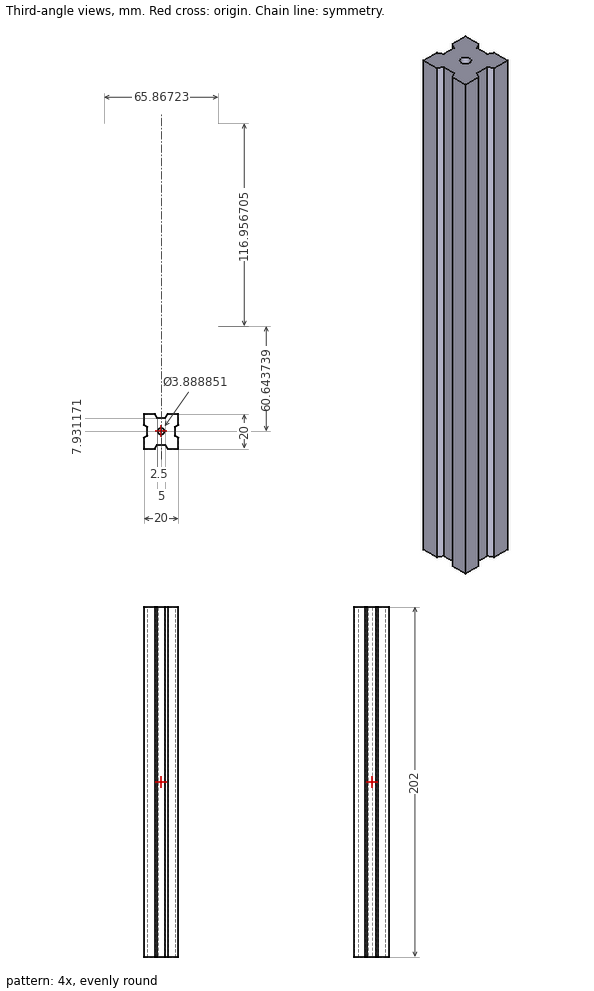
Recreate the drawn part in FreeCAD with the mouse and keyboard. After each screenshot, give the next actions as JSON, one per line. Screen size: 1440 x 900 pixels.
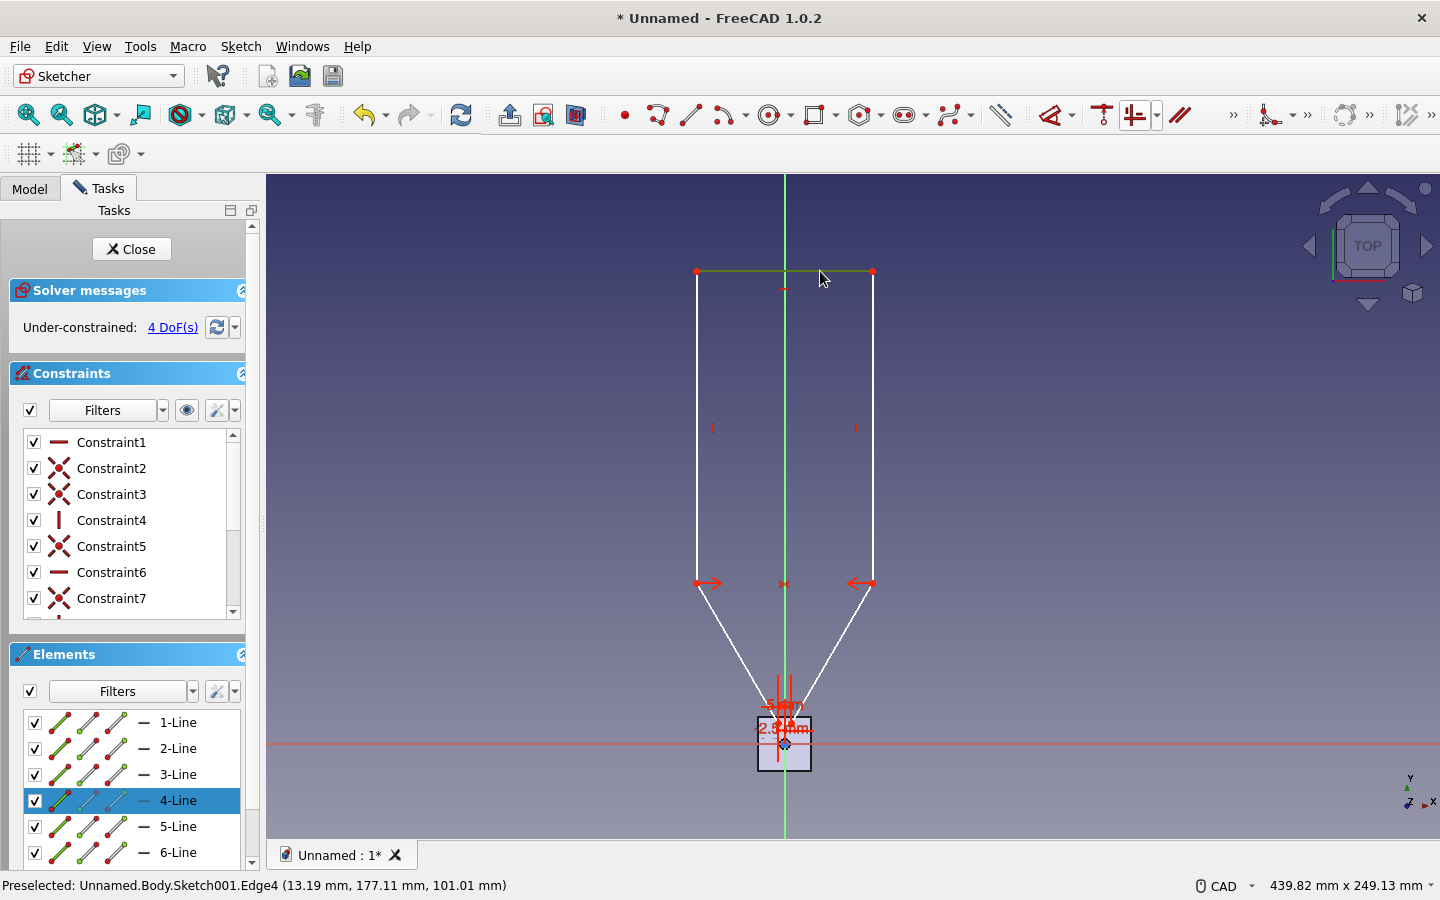
{"action": "key", "text": "l"}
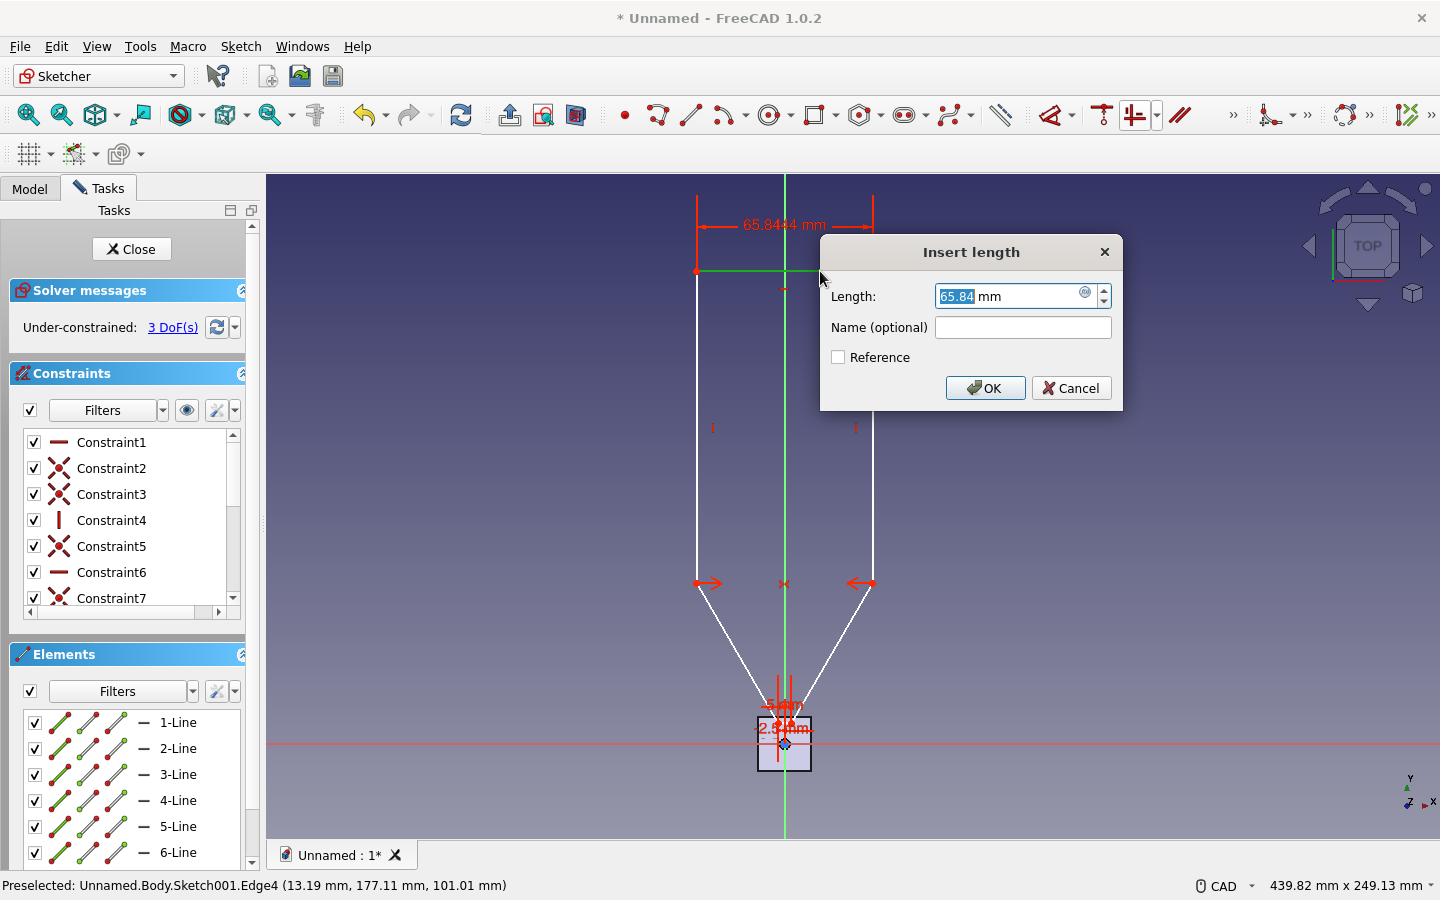
{"action": "type", "text": "65.86723"}
{"action": "key", "text": "Return"}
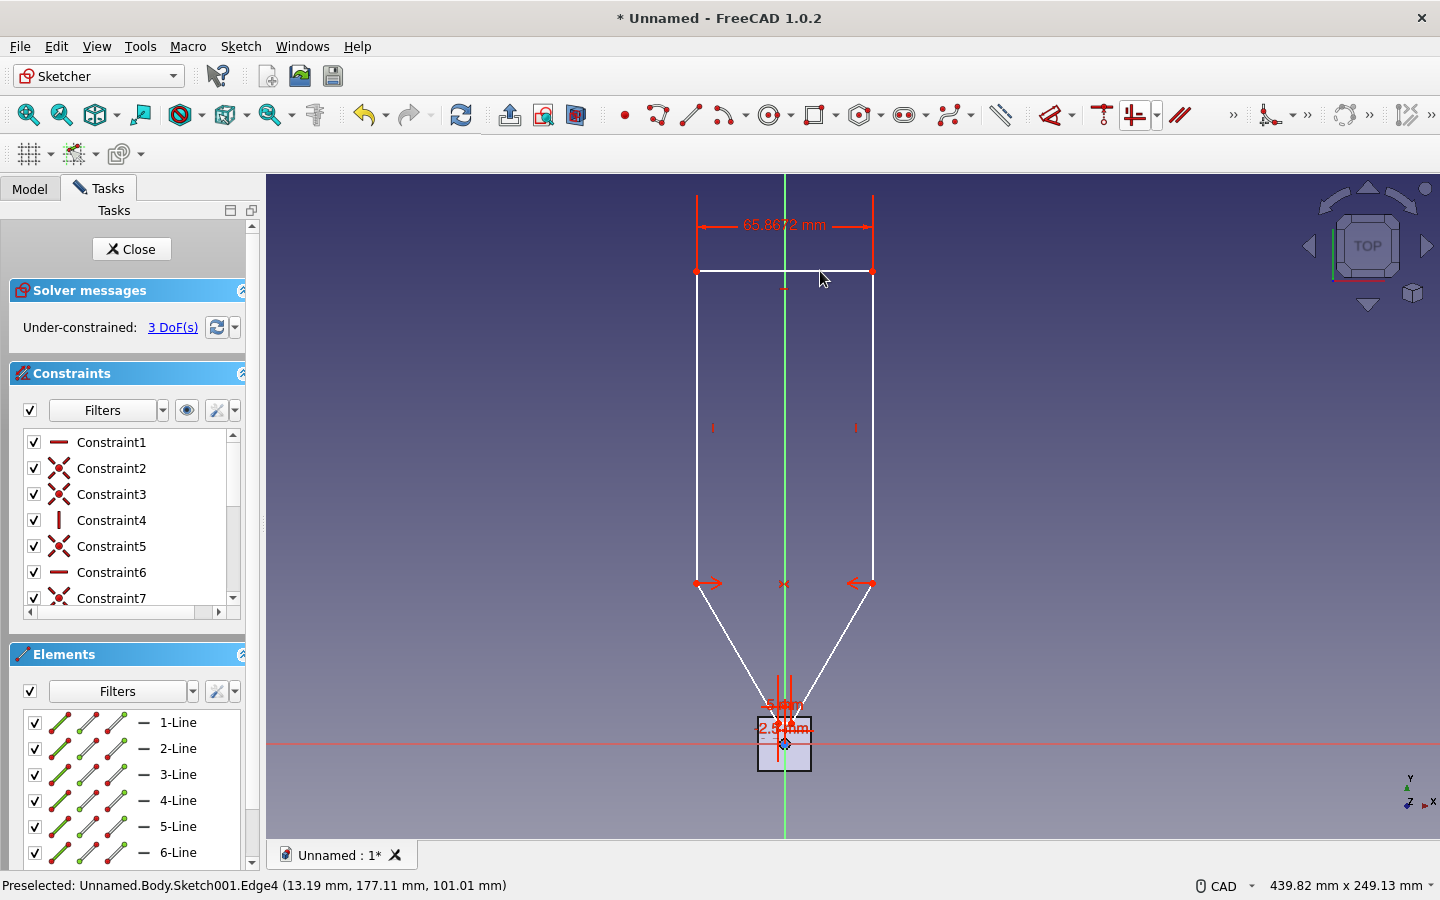
{"action": "scroll", "coordinate": [778, 723], "scroll_direction": "up", "scroll_amount": 4}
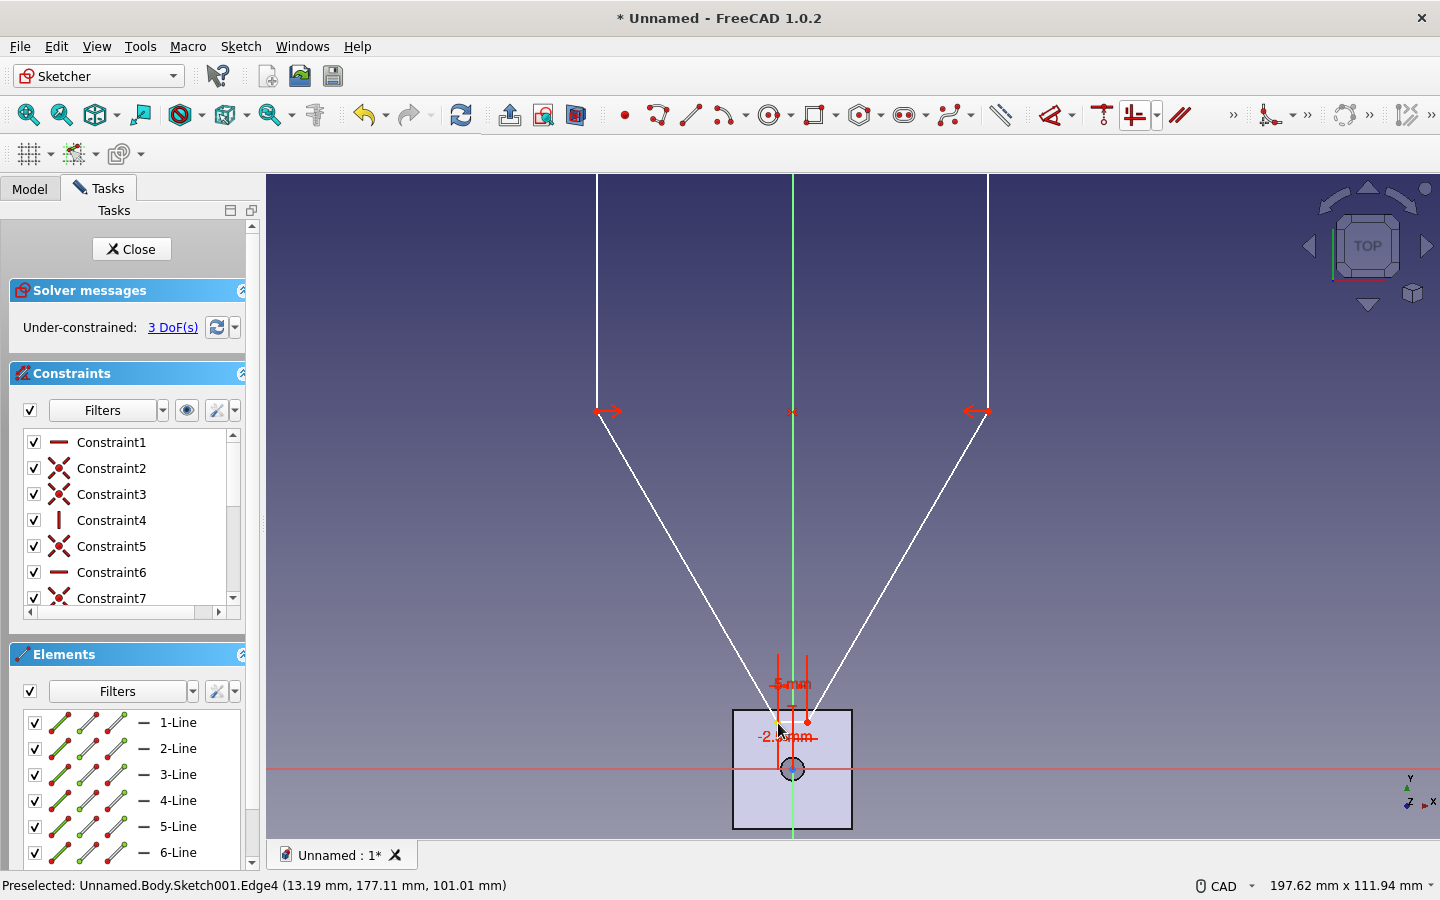
{"action": "left_click", "coordinate": [778, 722]}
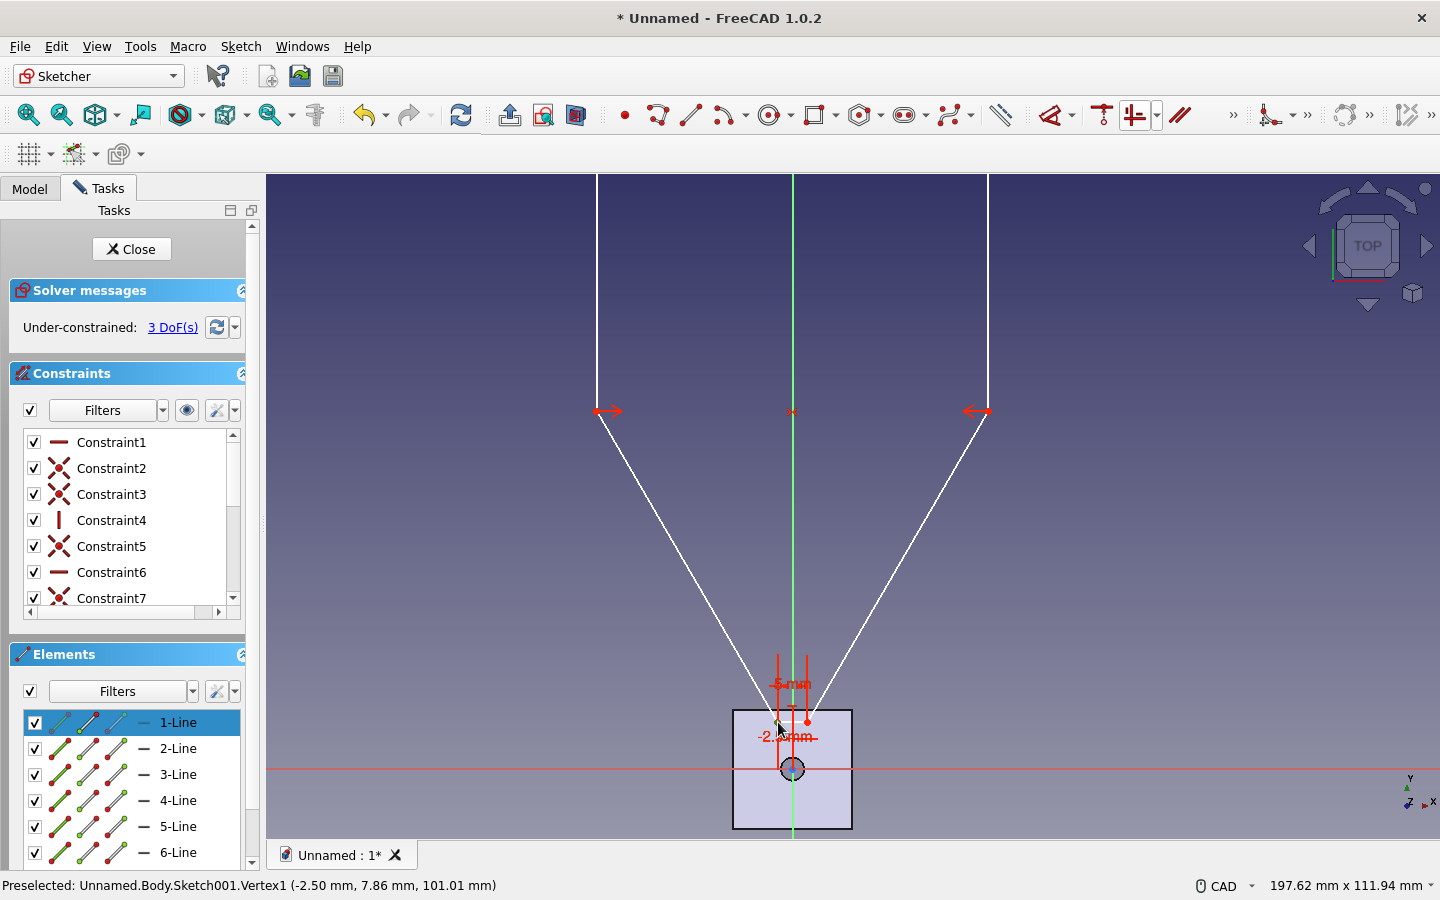
{"action": "key", "text": "i"}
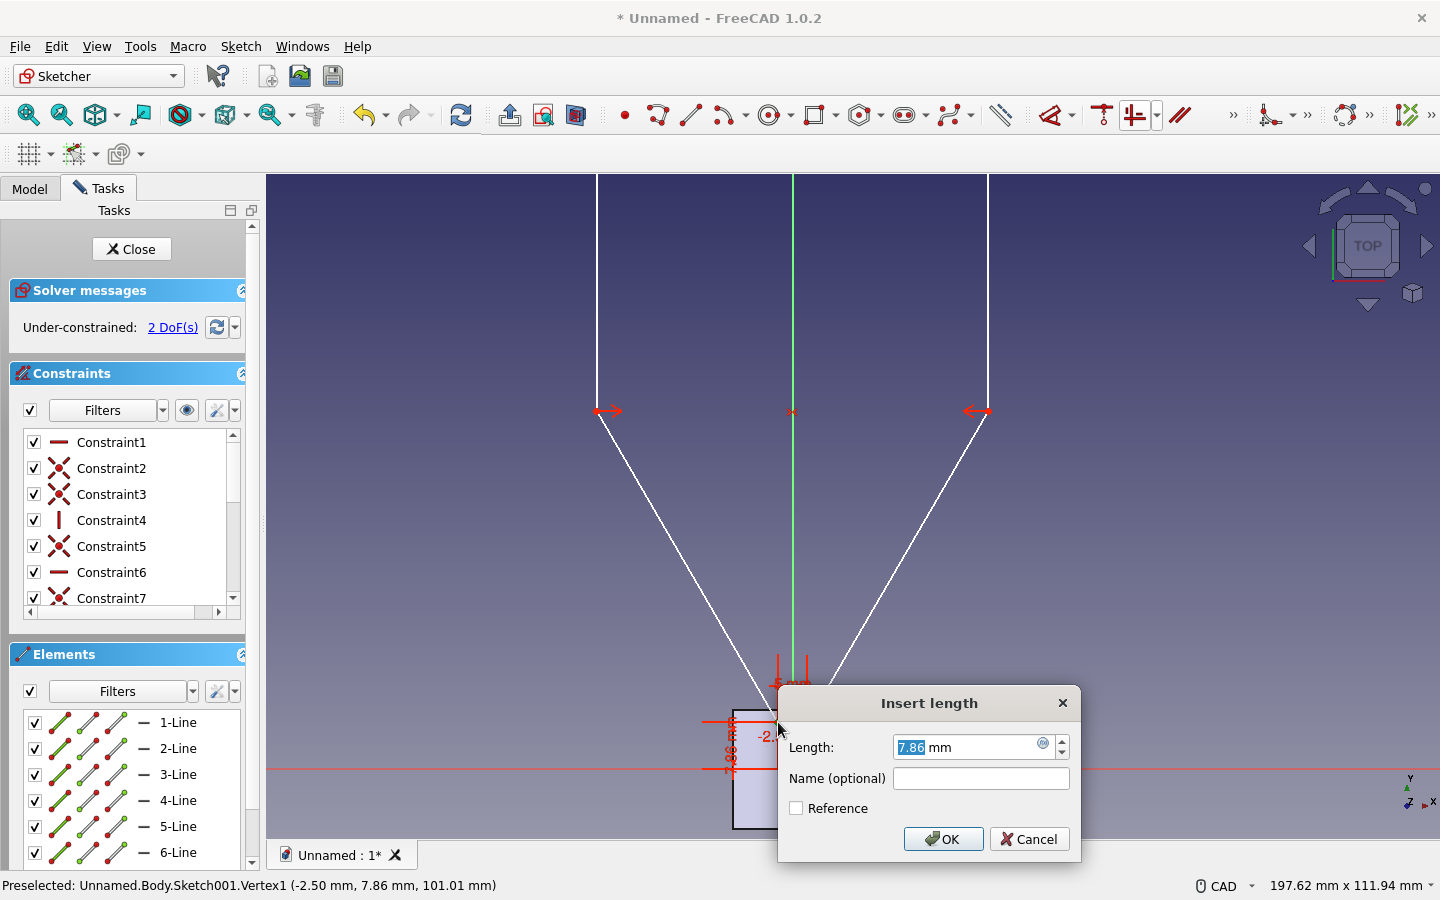
{"action": "type", "text": "7.931171"}
{"action": "key", "text": "Return"}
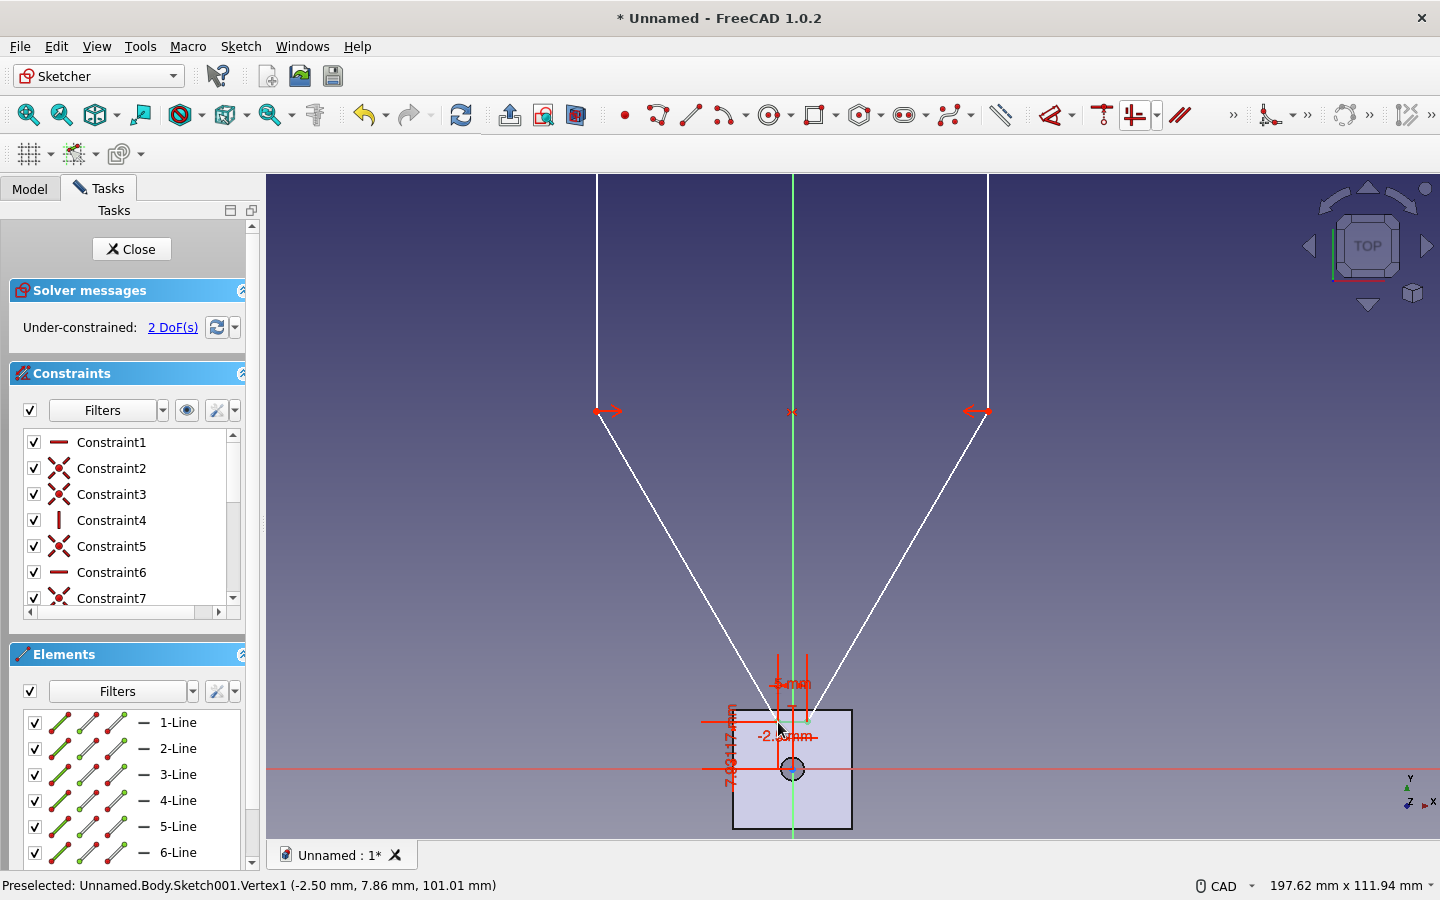
{"action": "left_click", "coordinate": [988, 203]}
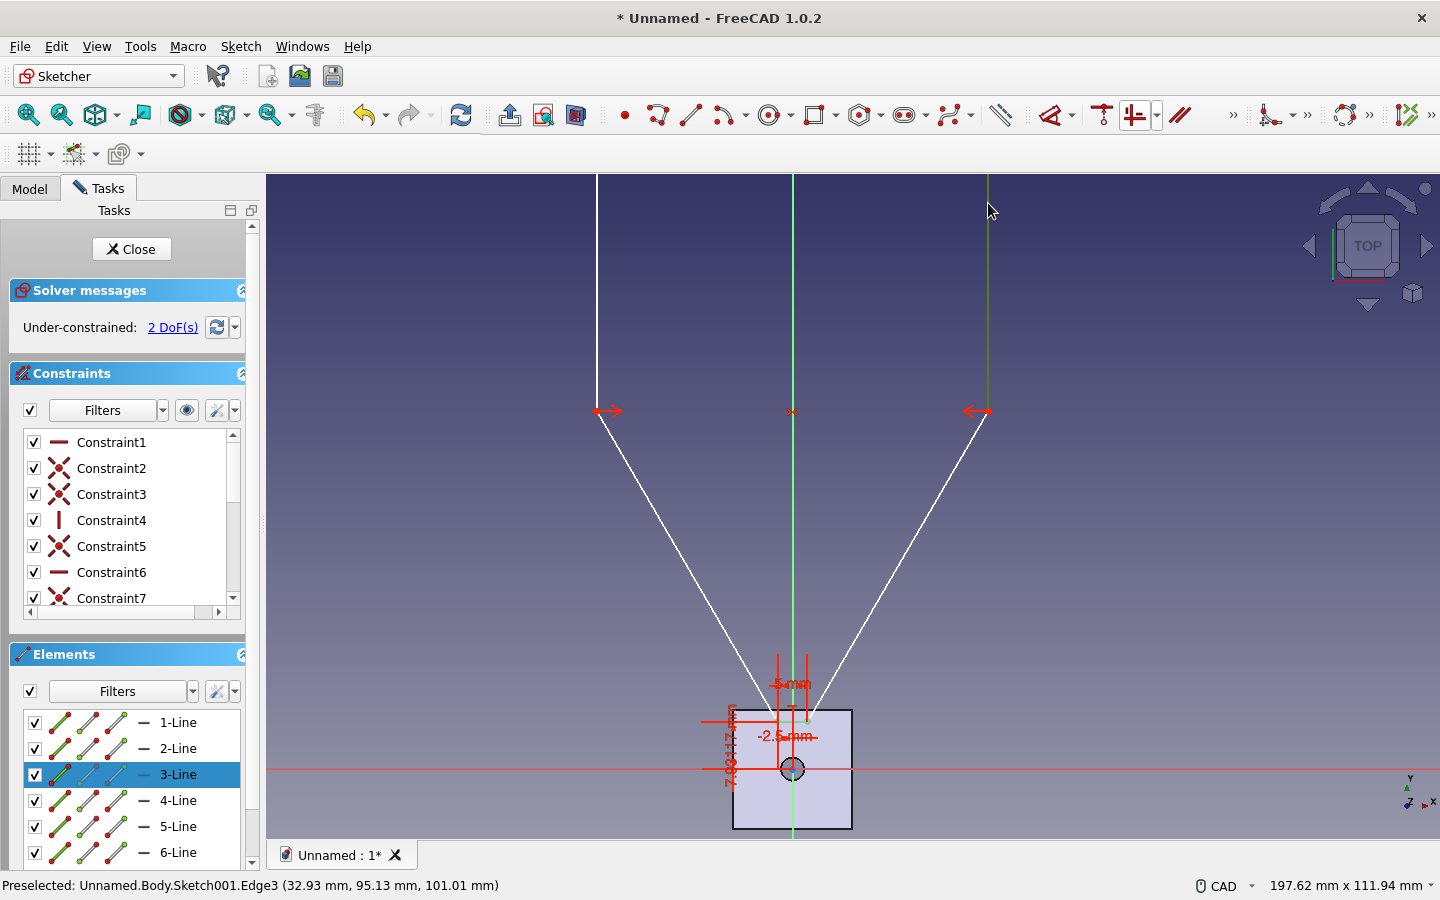
{"action": "key", "text": "i"}